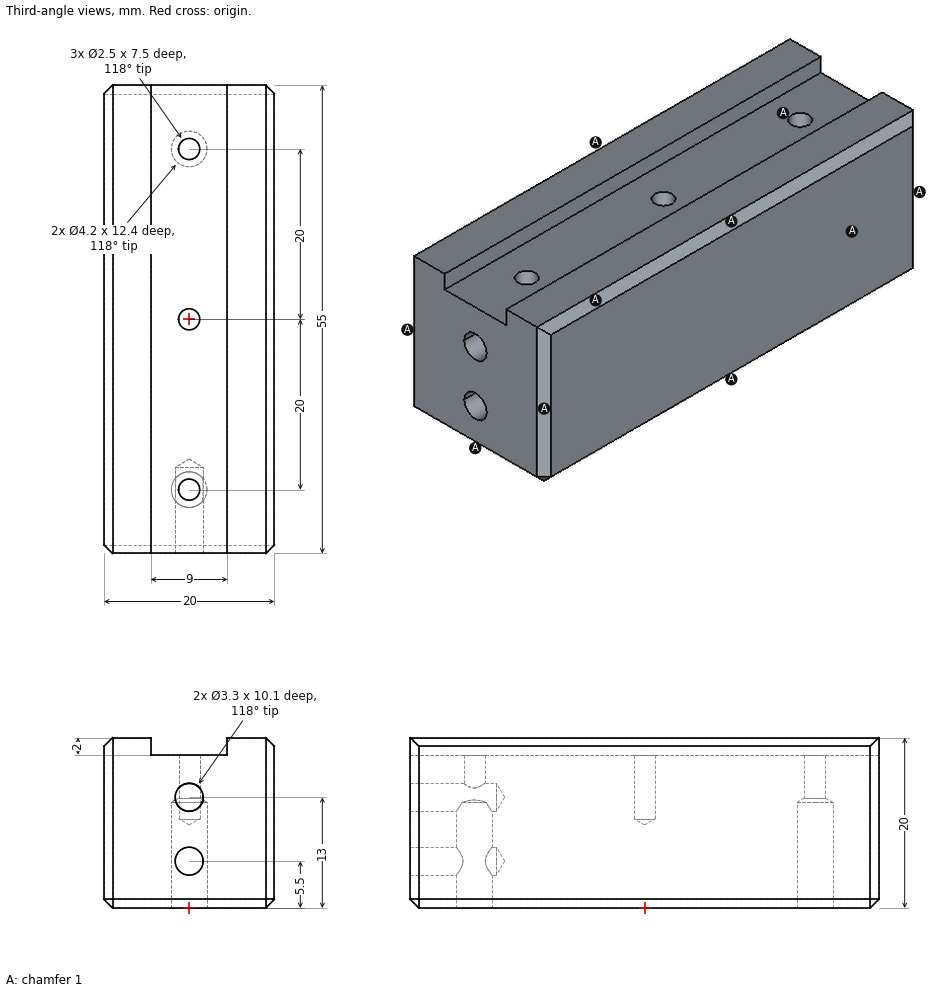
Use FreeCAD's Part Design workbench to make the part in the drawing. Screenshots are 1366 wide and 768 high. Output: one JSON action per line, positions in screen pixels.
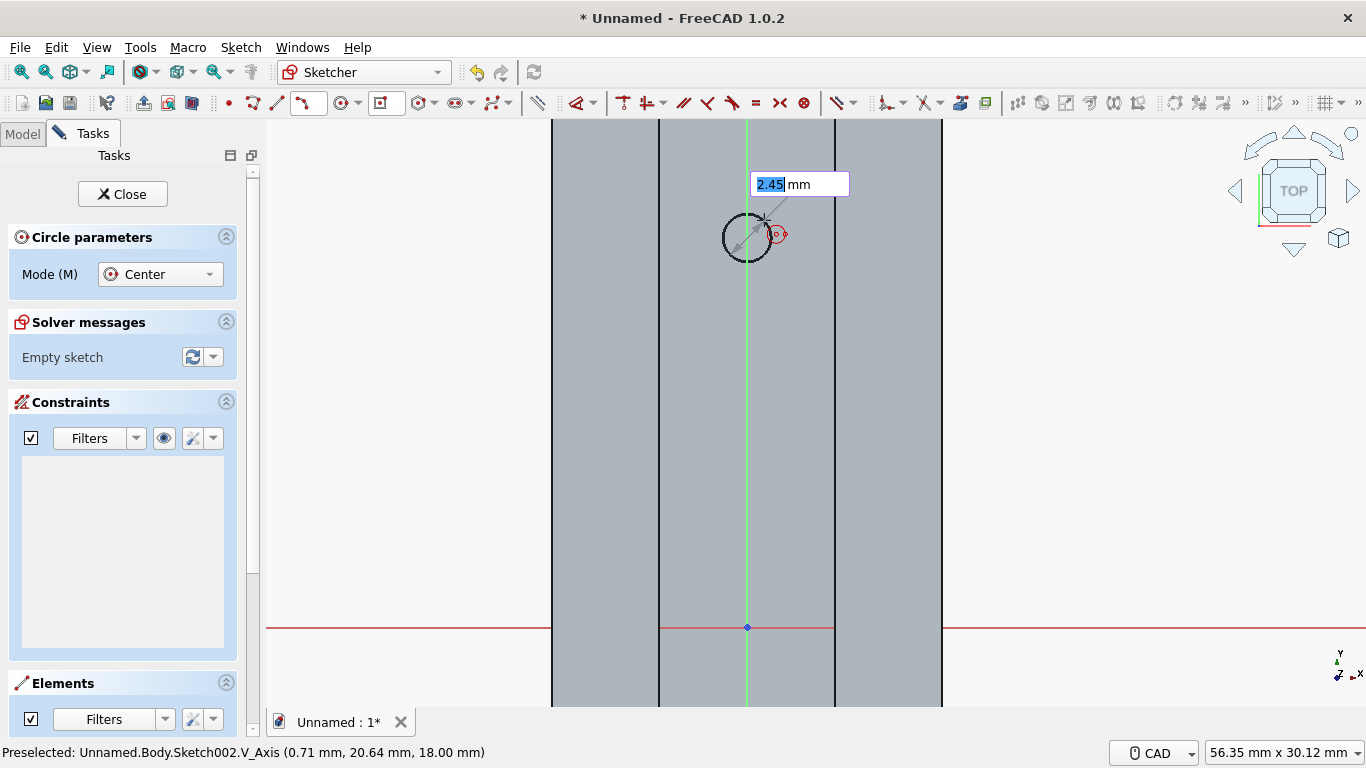
{"action": "type", "text": "2.5"}
{"action": "key", "text": "Return"}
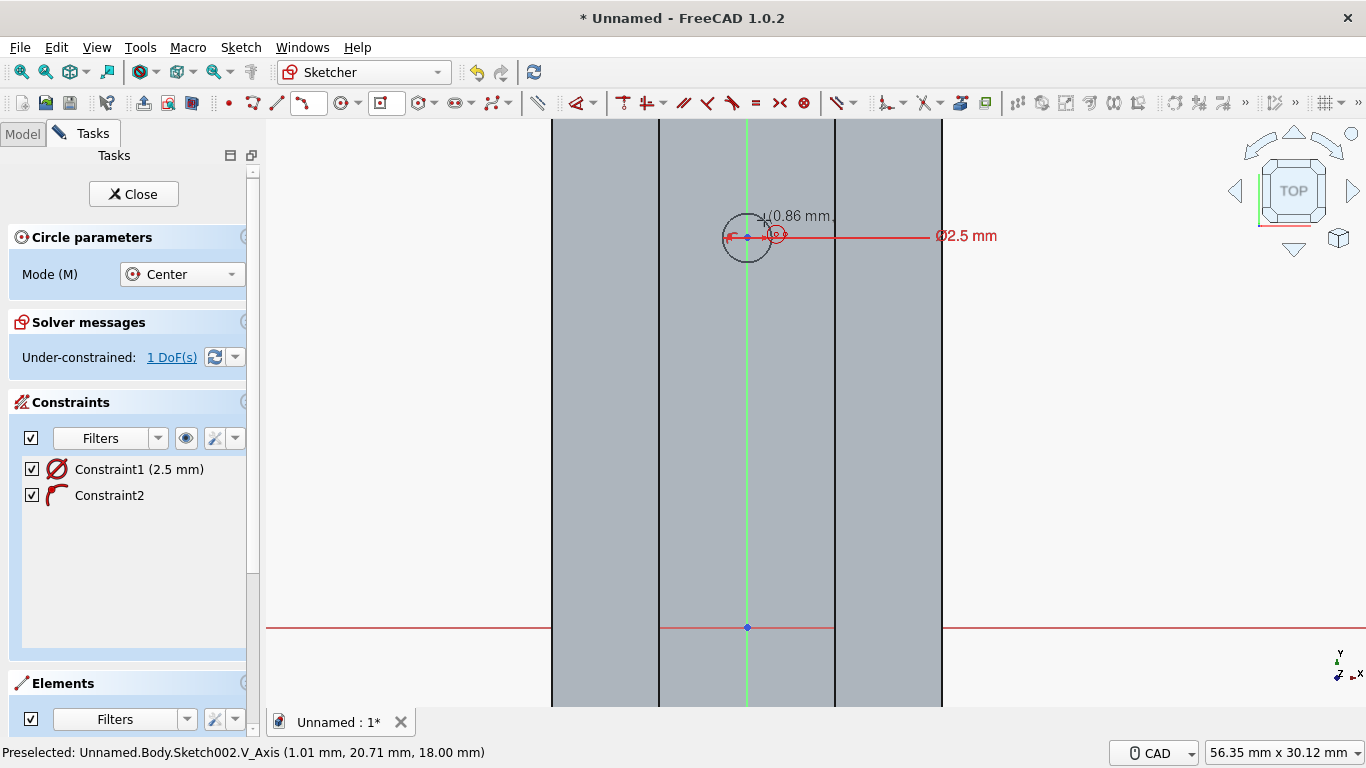
{"action": "left_click", "coordinate": [747, 628]}
{"action": "mouse_move", "coordinate": [764, 611]}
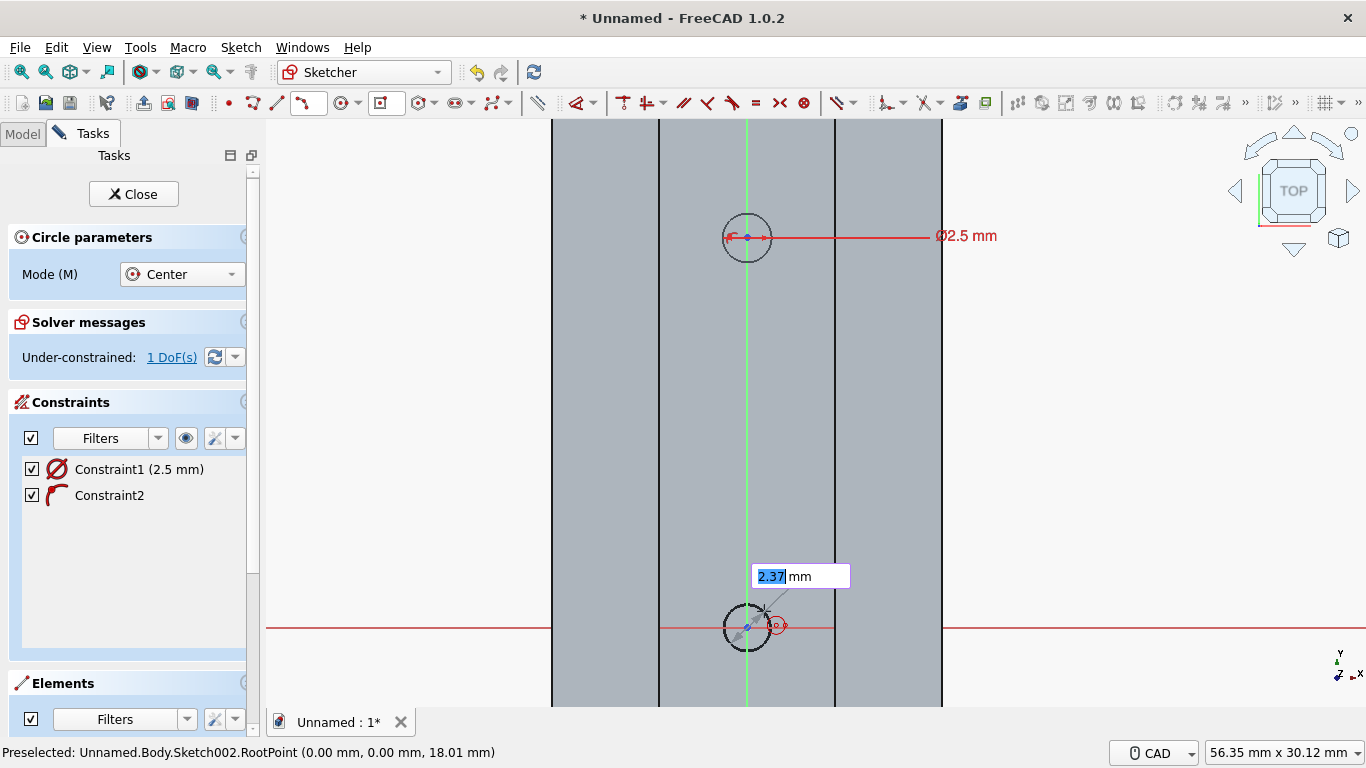
{"action": "type", "text": "2.5"}
{"action": "key", "text": "Return"}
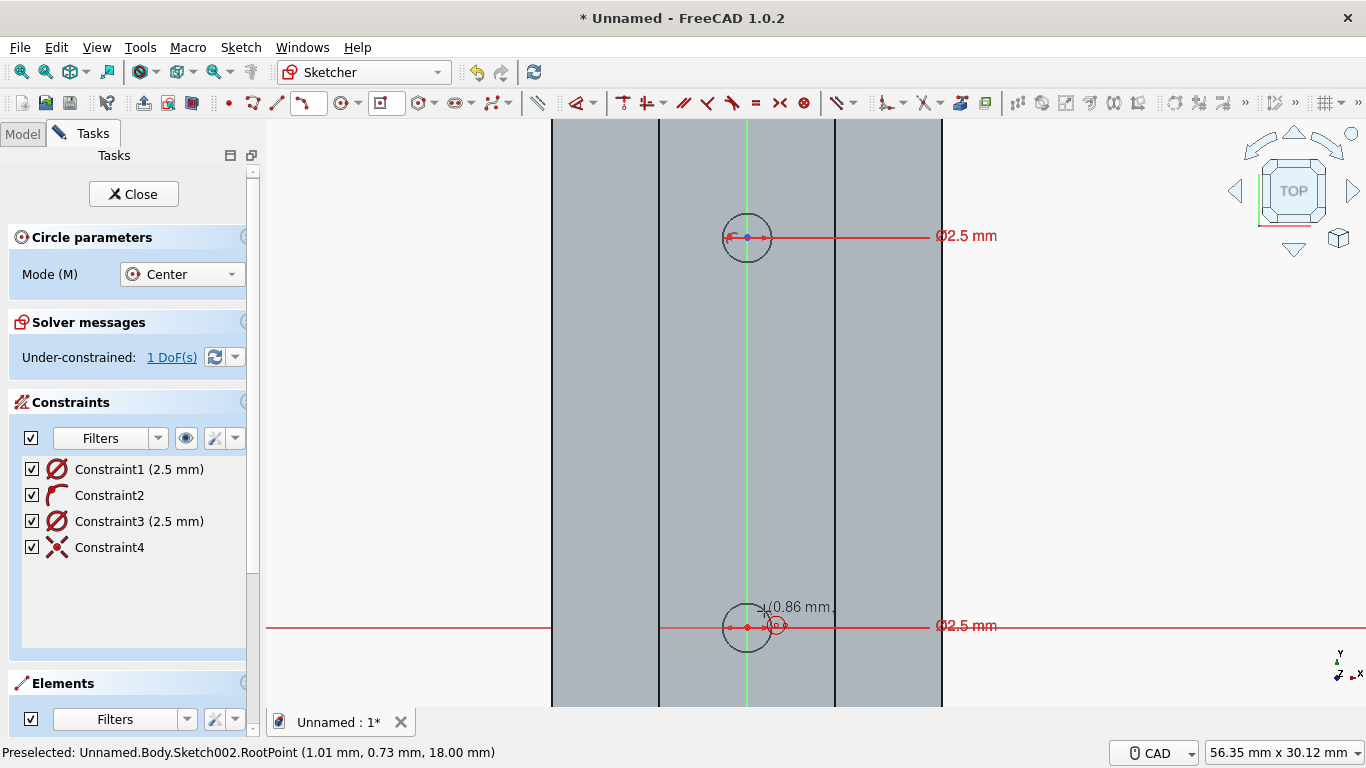
{"action": "scroll", "coordinate": [748, 238], "scroll_direction": "down", "scroll_amount": 4}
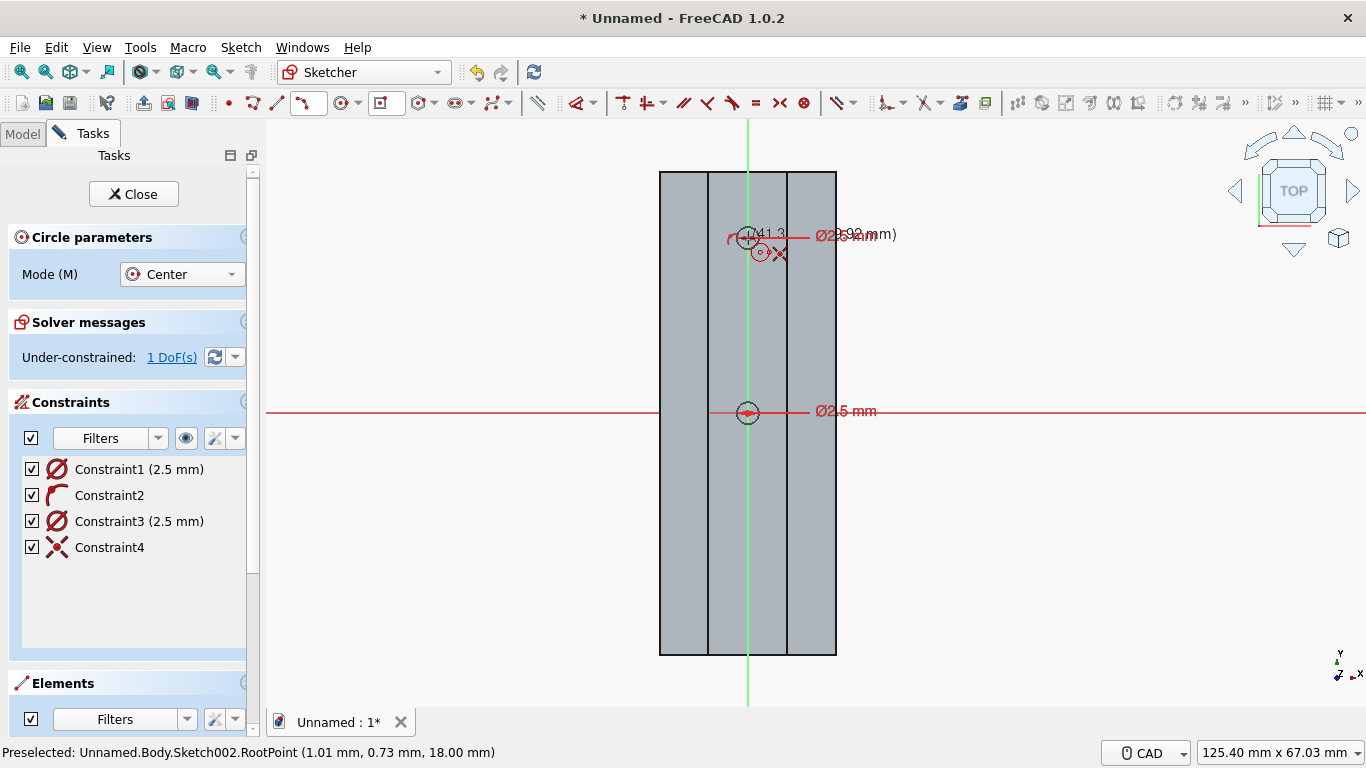
{"action": "scroll", "coordinate": [748, 589], "scroll_direction": "up", "scroll_amount": 4}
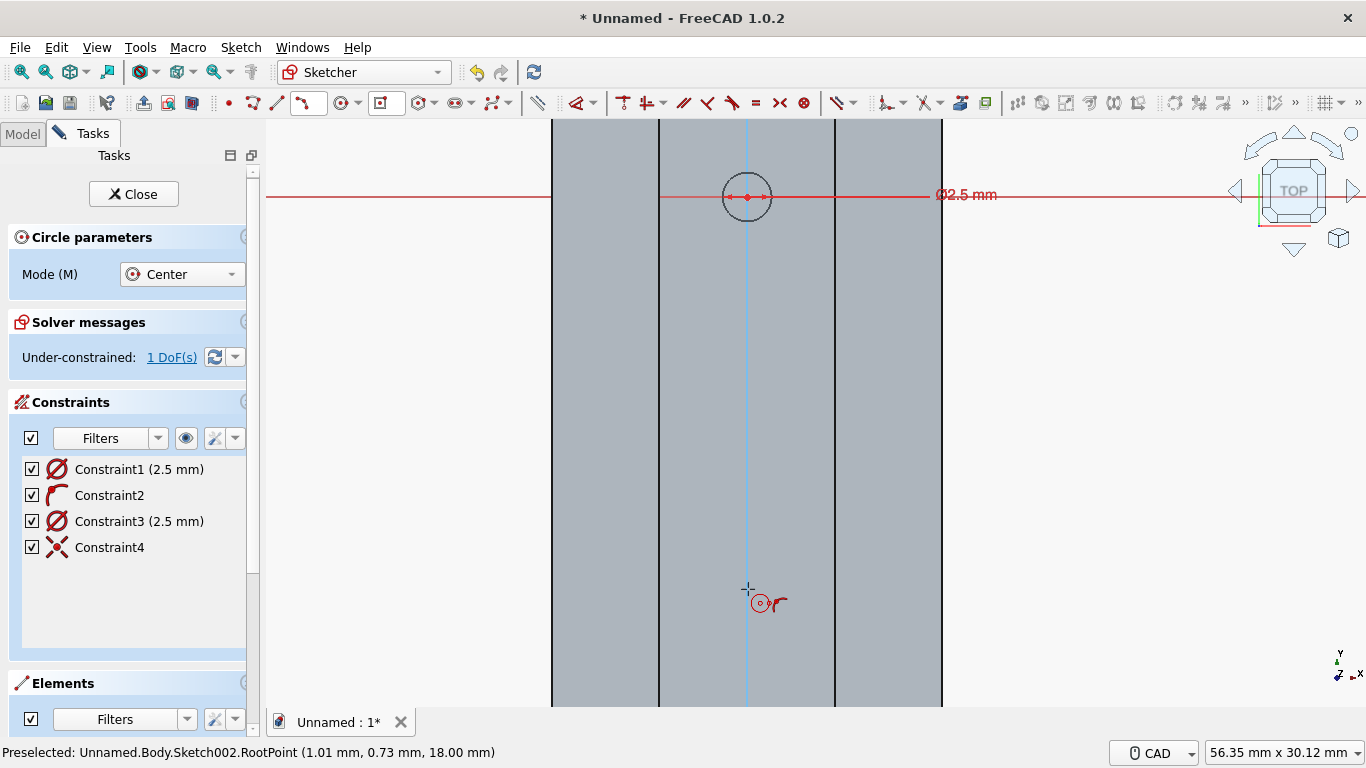
{"action": "left_click", "coordinate": [747, 587]}
{"action": "mouse_move", "coordinate": [764, 570]}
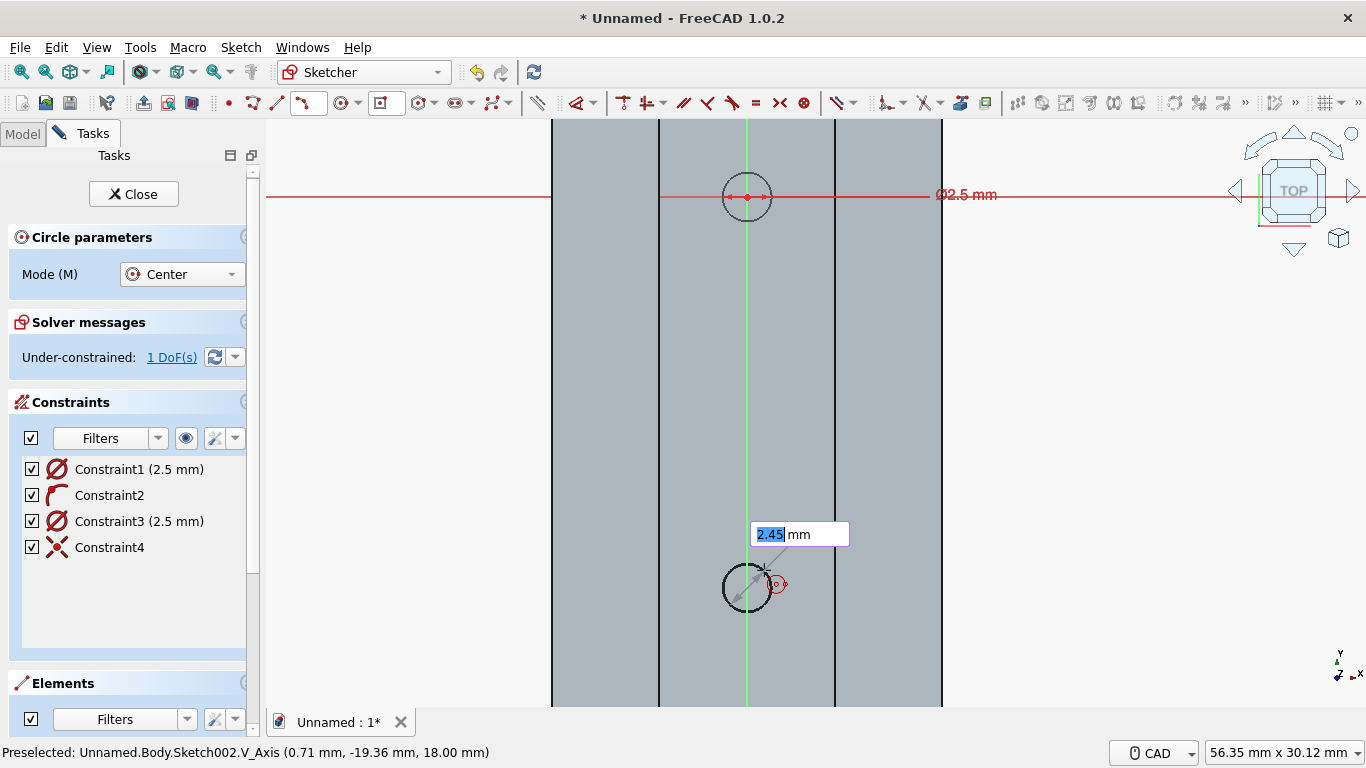
{"action": "type", "text": "2.5"}
{"action": "key", "text": "Return"}
{"action": "key", "text": "Escape"}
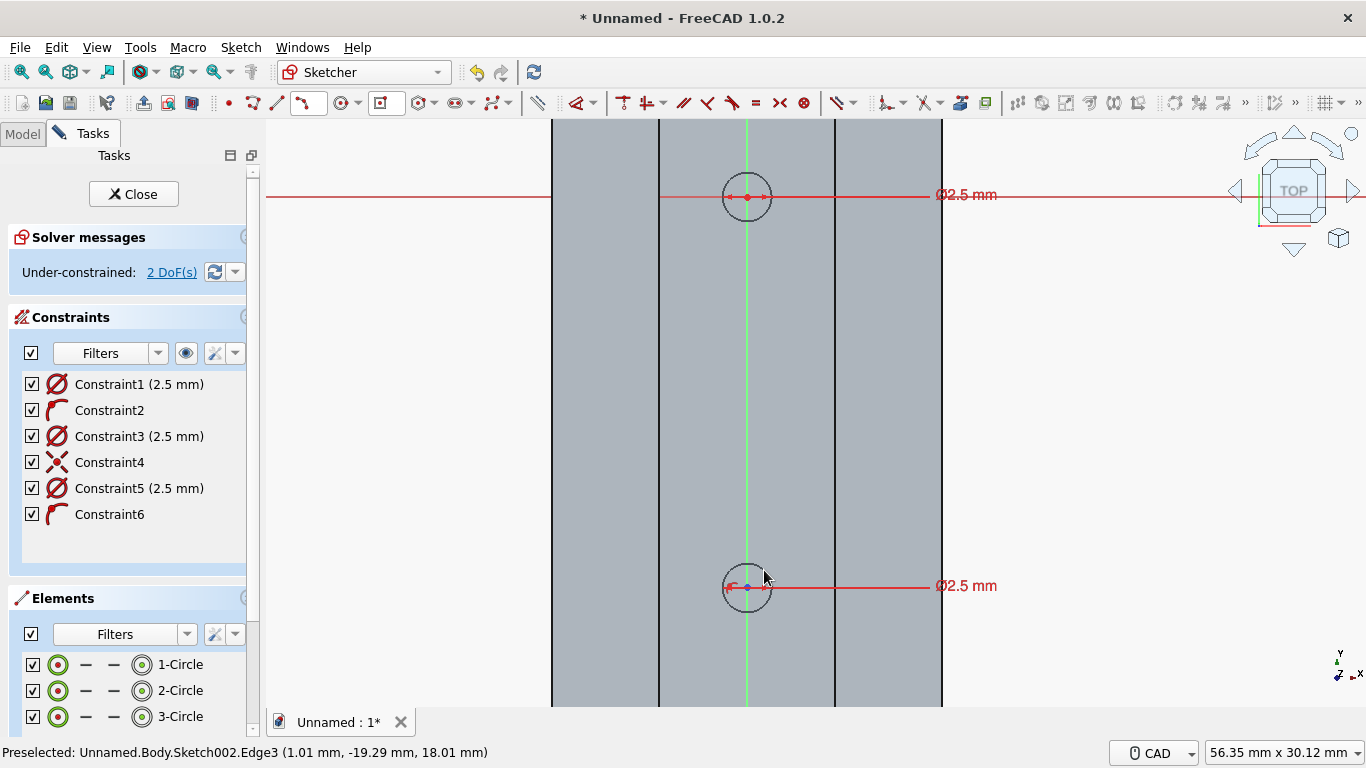
{"action": "left_click", "coordinate": [576, 104]}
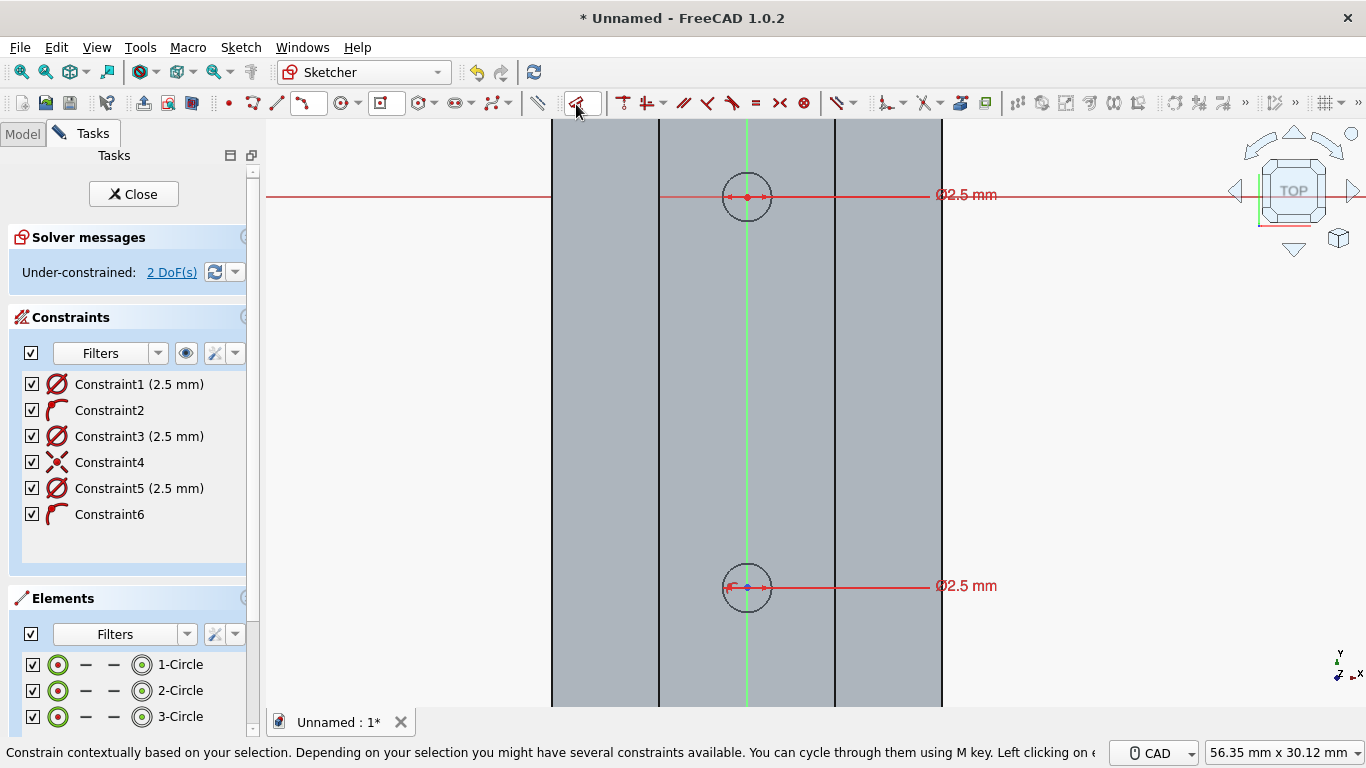
{"action": "scroll", "coordinate": [748, 589], "scroll_direction": "down", "scroll_amount": 4}